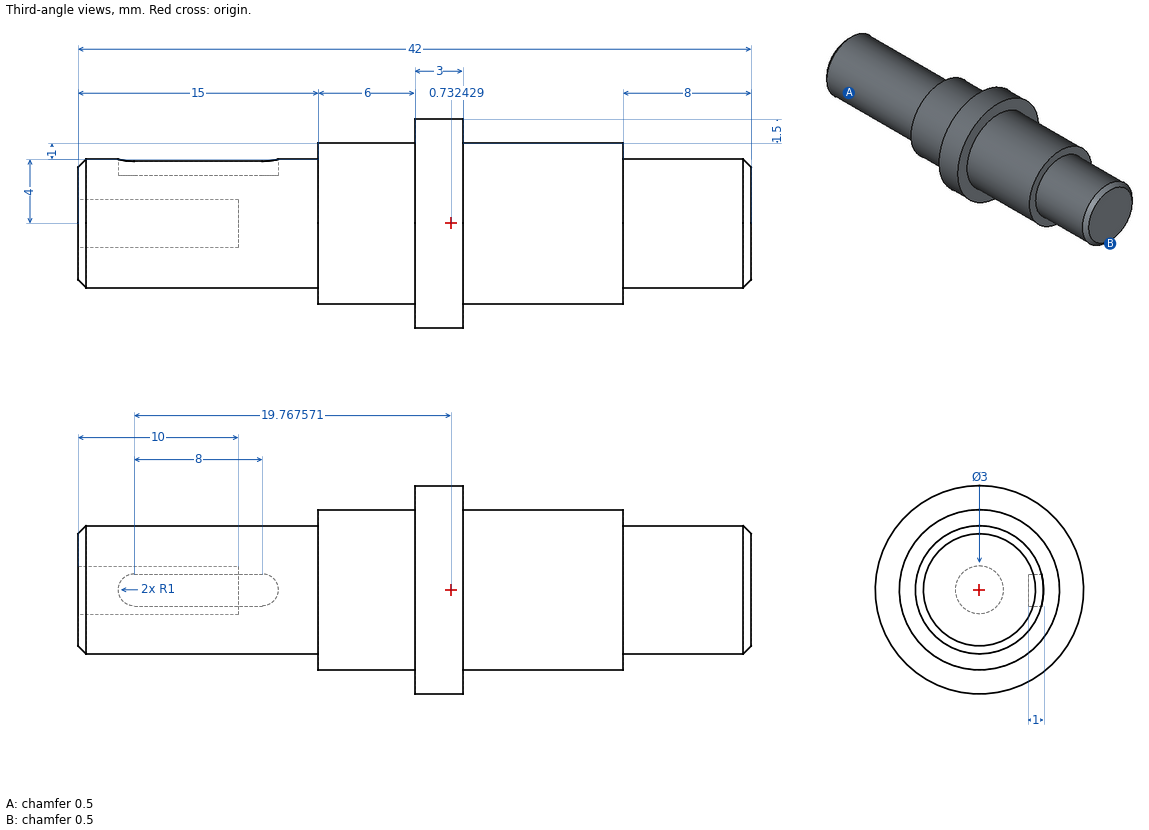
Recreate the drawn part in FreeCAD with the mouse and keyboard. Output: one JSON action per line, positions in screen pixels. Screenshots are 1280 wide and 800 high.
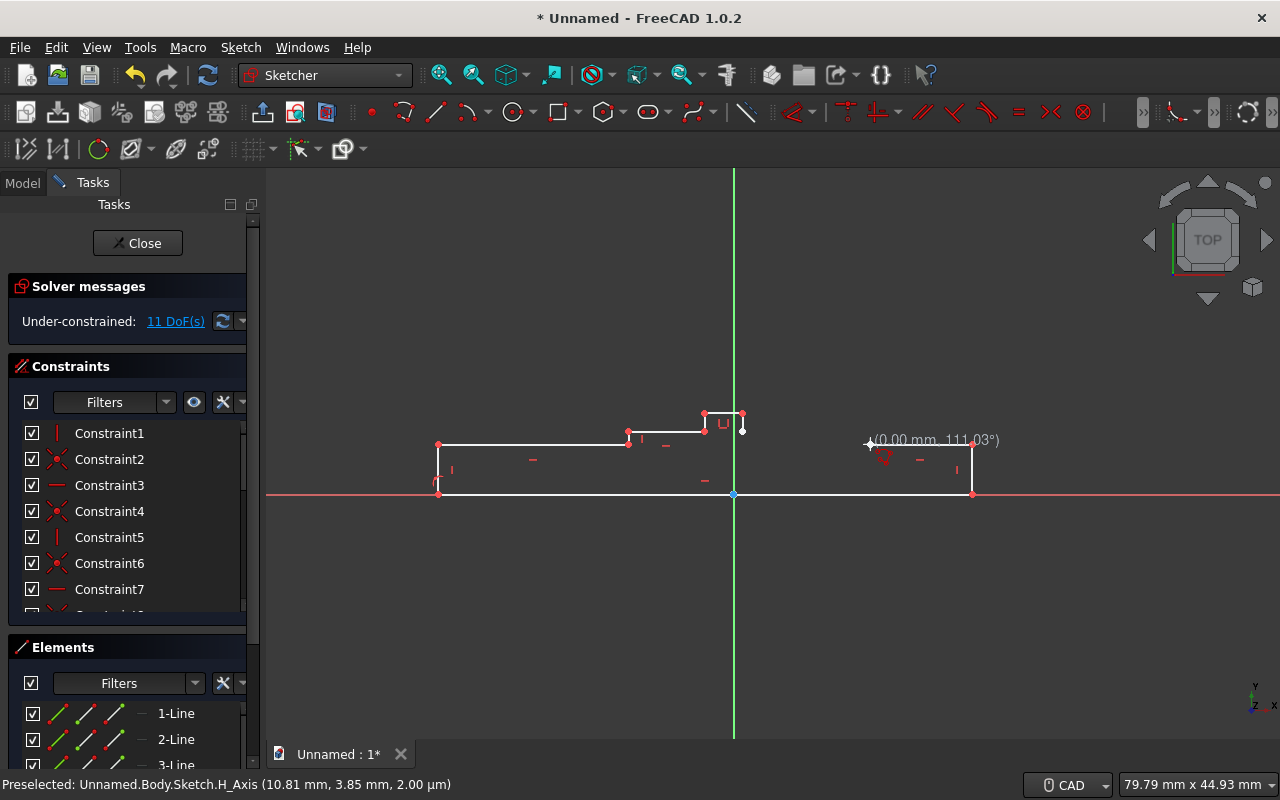
{"action": "scroll", "coordinate": [870, 431], "scroll_direction": "up", "scroll_amount": 2}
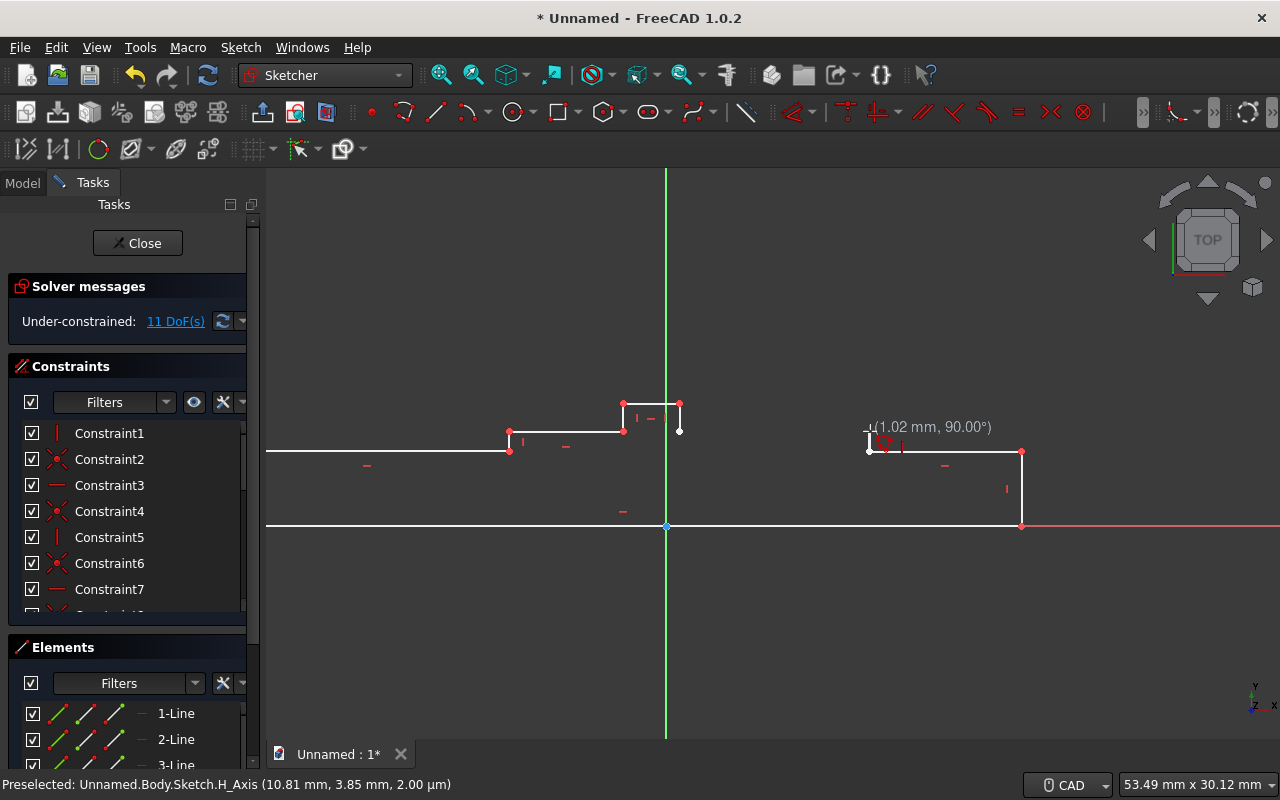
{"action": "left_click", "coordinate": [870, 431]}
{"action": "left_click", "coordinate": [680, 432]}
{"action": "key", "text": "Escape"}
{"action": "key", "text": "Escape"}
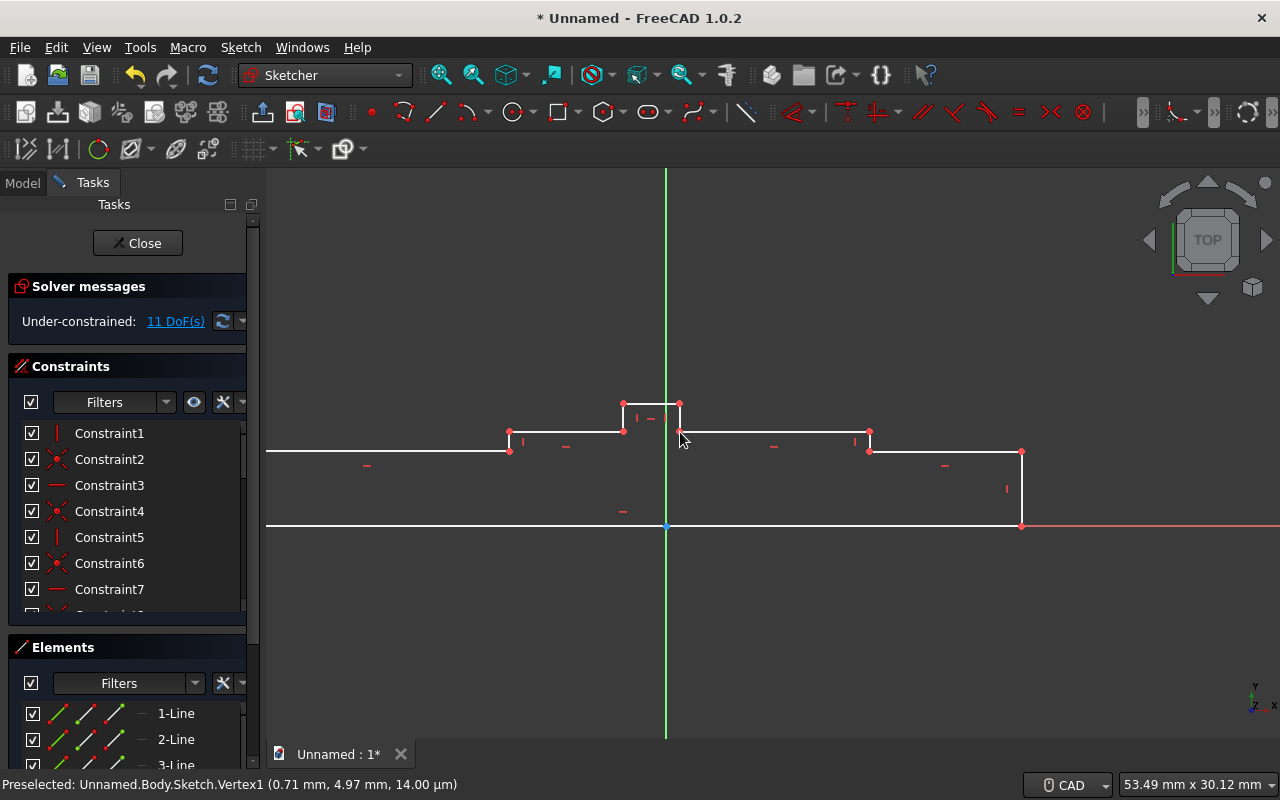
{"action": "left_click", "coordinate": [792, 112]}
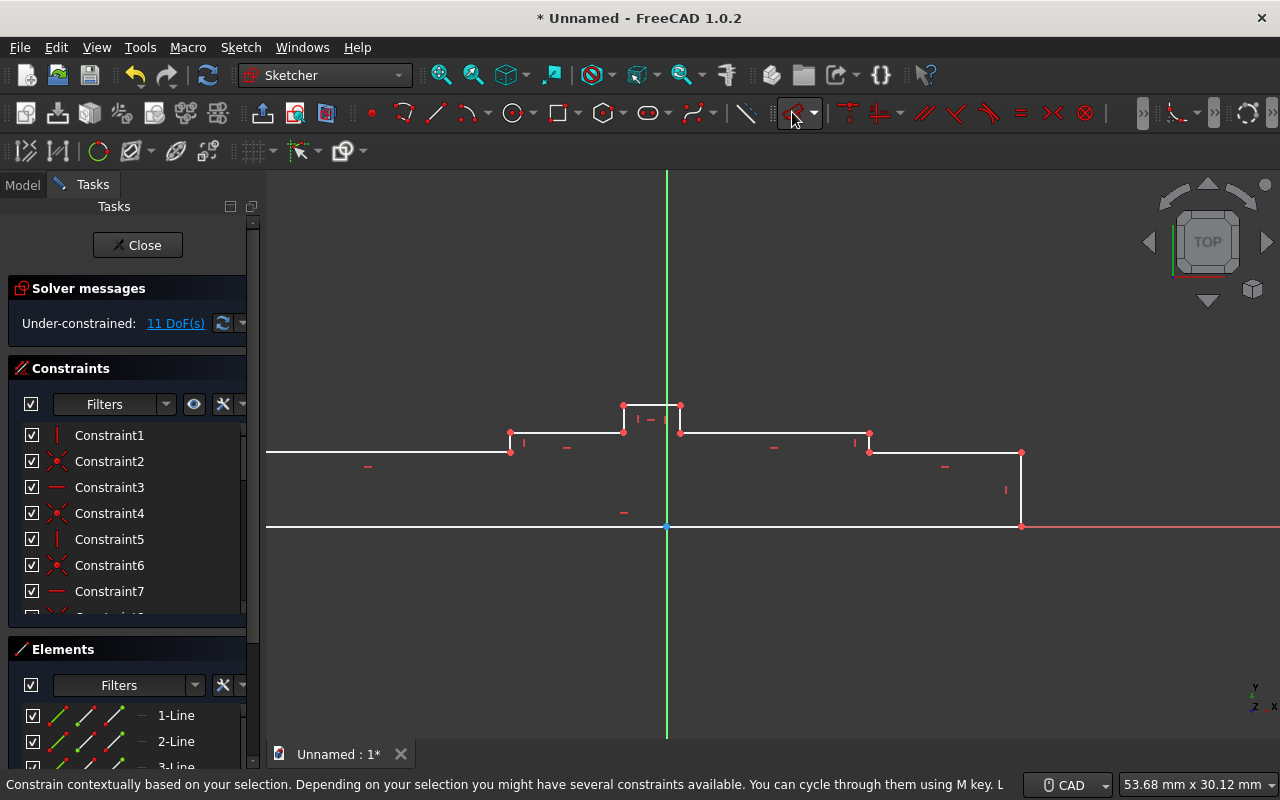
{"action": "left_click", "coordinate": [663, 405]}
{"action": "left_click", "coordinate": [652, 371]}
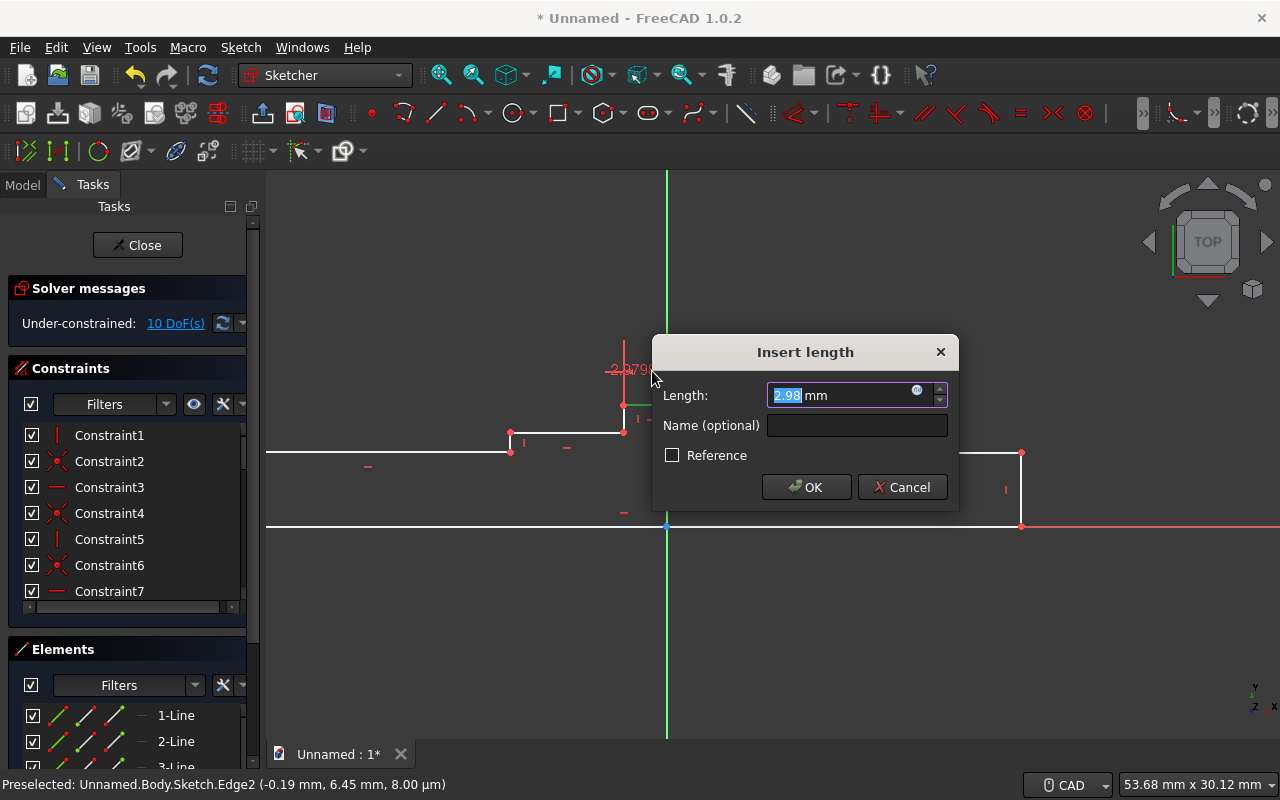
{"action": "type", "text": "3"}
{"action": "key", "text": "Return"}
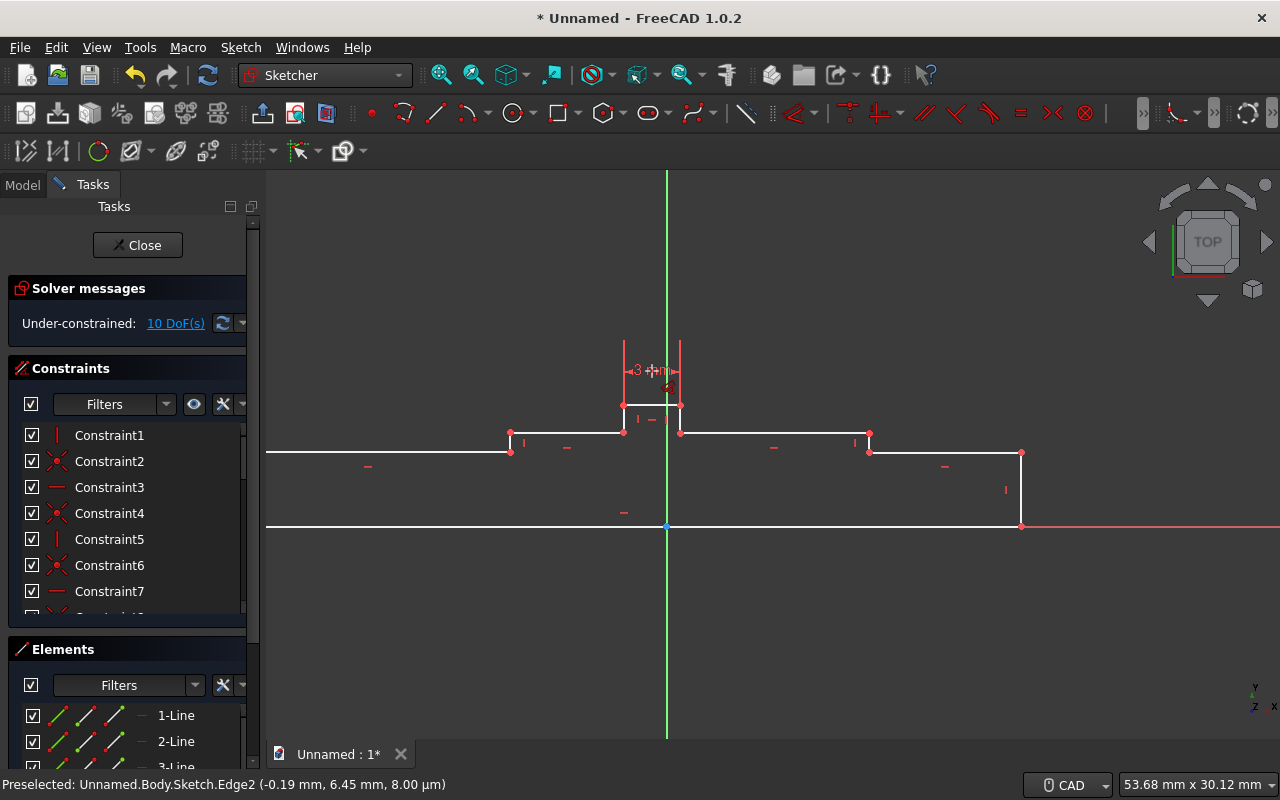
{"action": "left_click", "coordinate": [590, 433]}
{"action": "left_click", "coordinate": [567, 399]}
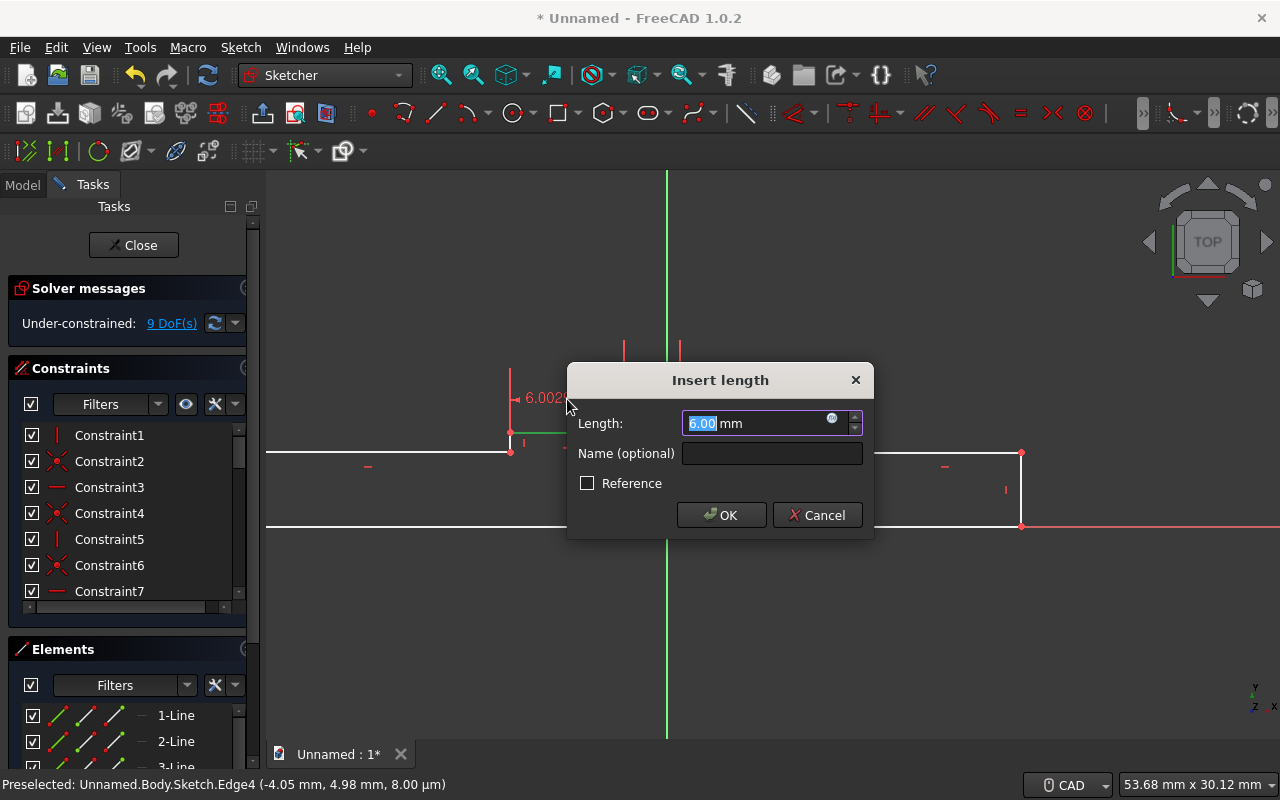
{"action": "type", "text": "6"}
{"action": "key", "text": "Return"}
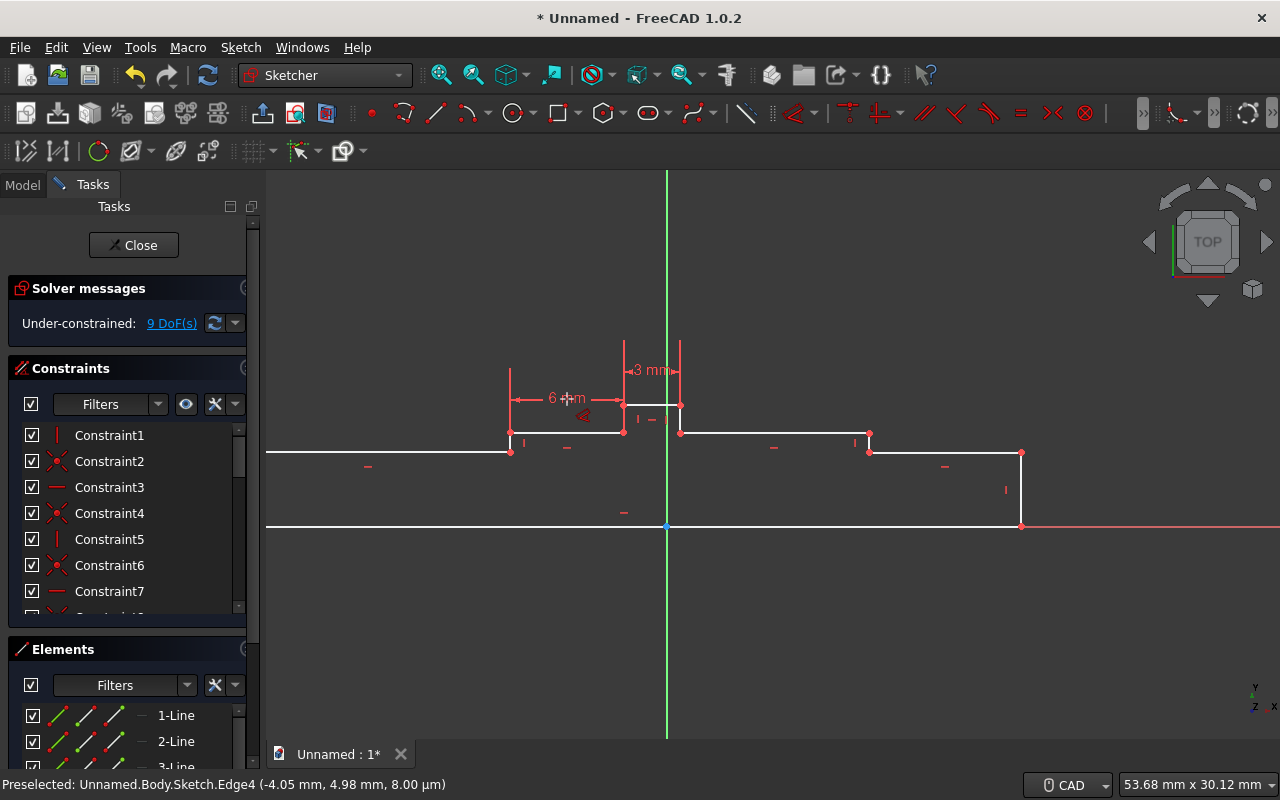
{"action": "scroll", "coordinate": [510, 443], "scroll_direction": "up", "scroll_amount": 4}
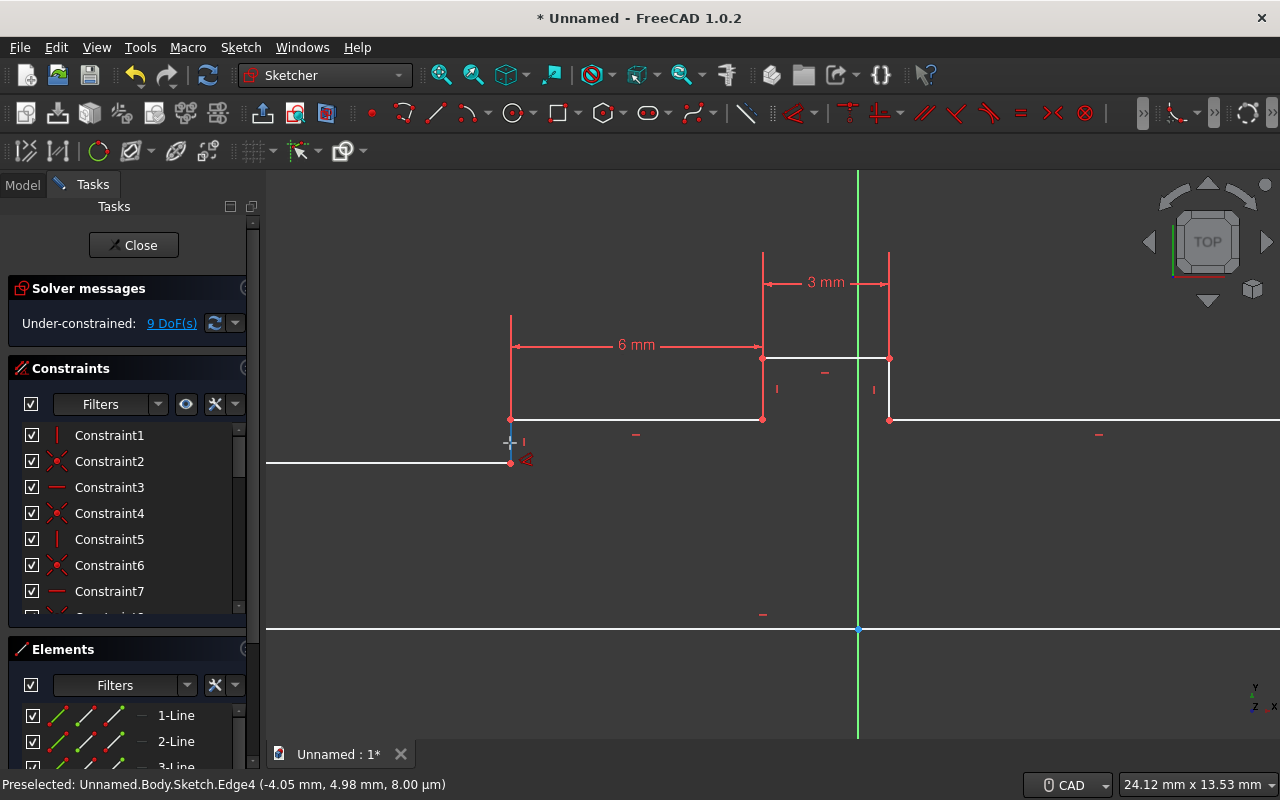
{"action": "left_click", "coordinate": [511, 442]}
{"action": "left_click", "coordinate": [477, 442]}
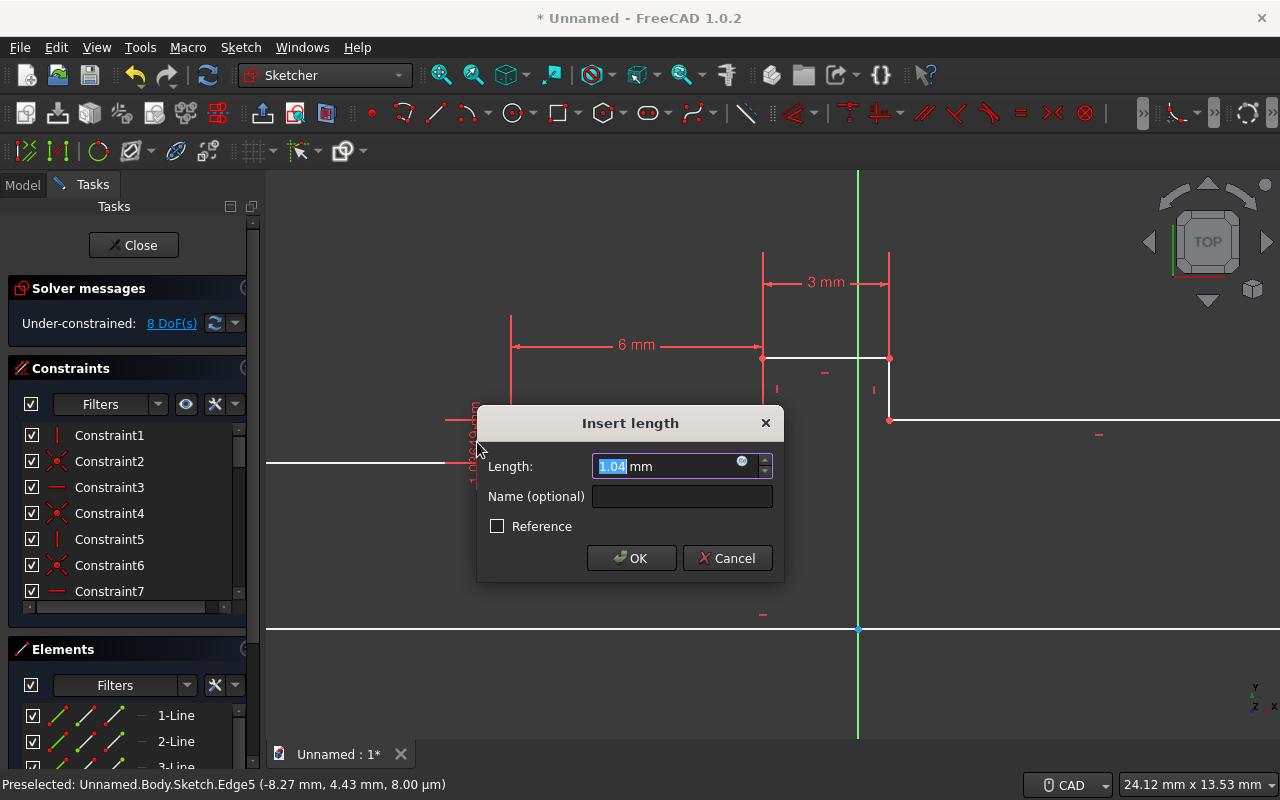
{"action": "type", "text": "1"}
{"action": "key", "text": "Return"}